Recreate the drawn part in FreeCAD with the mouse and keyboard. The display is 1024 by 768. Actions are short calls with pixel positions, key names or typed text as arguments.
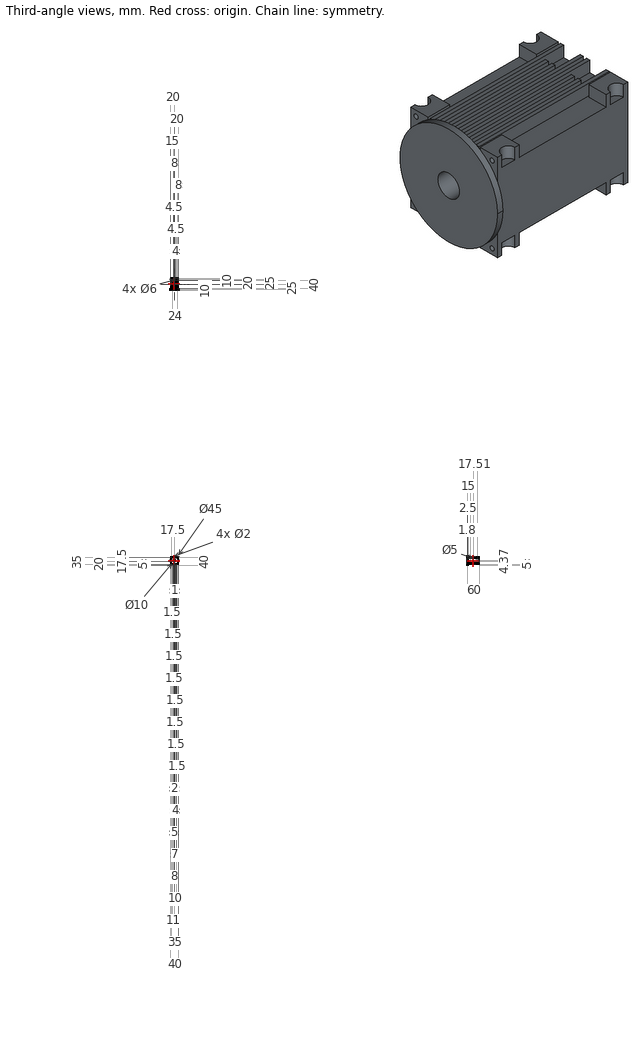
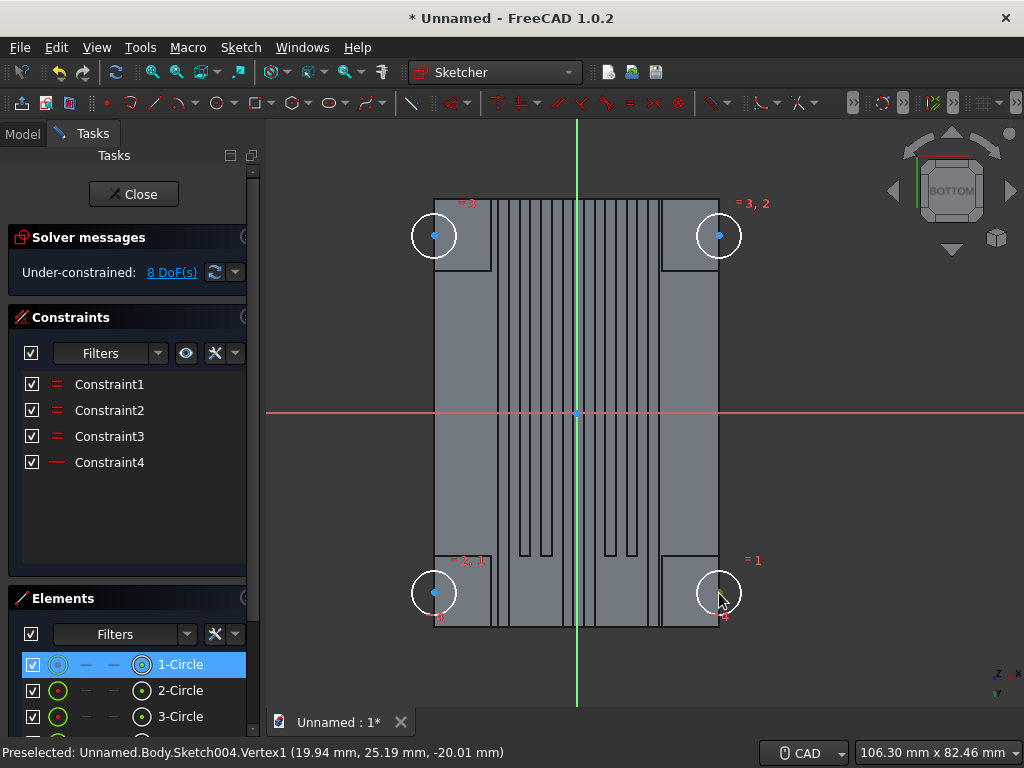
click(719, 236)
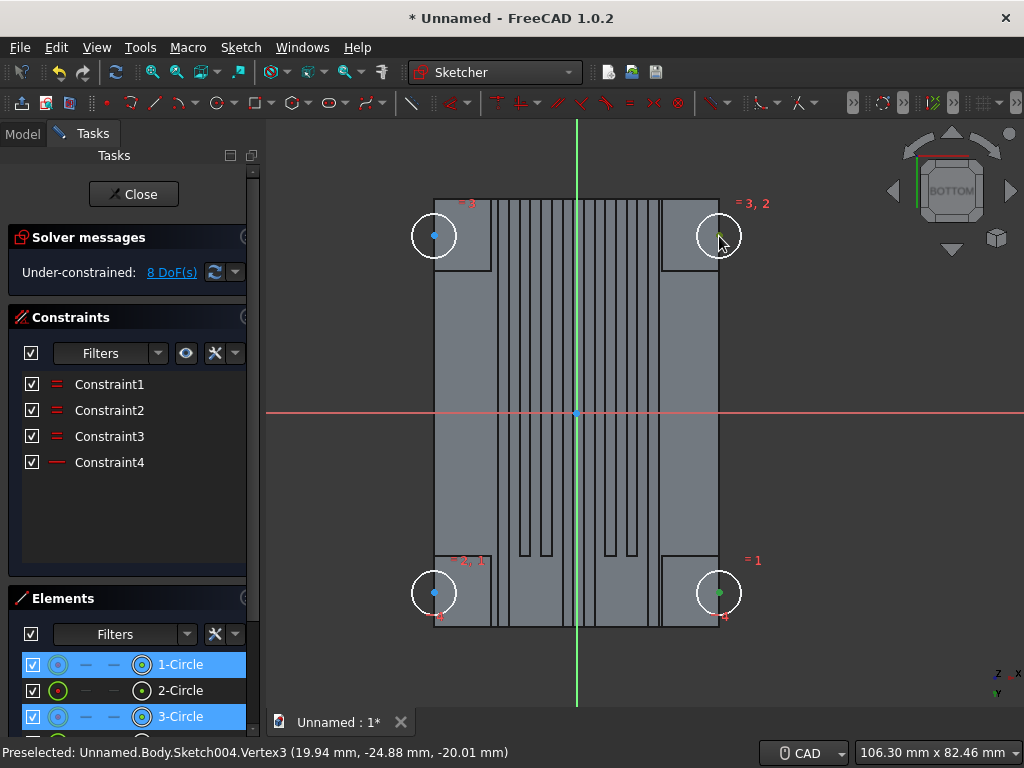
click(540, 104)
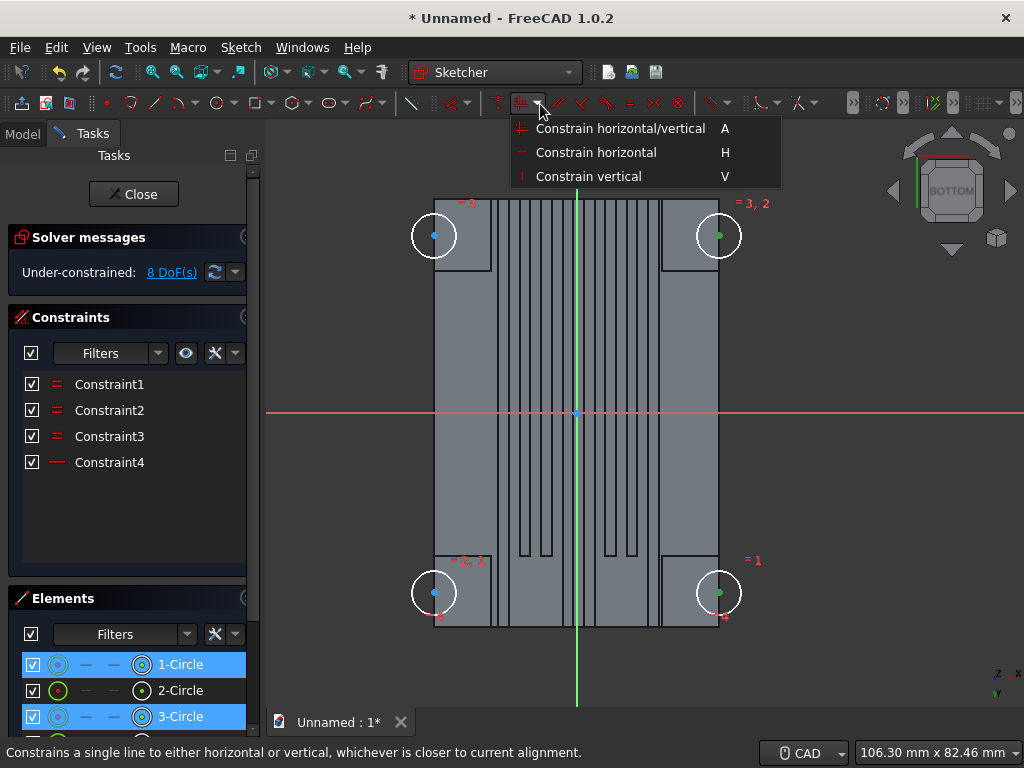
click(646, 176)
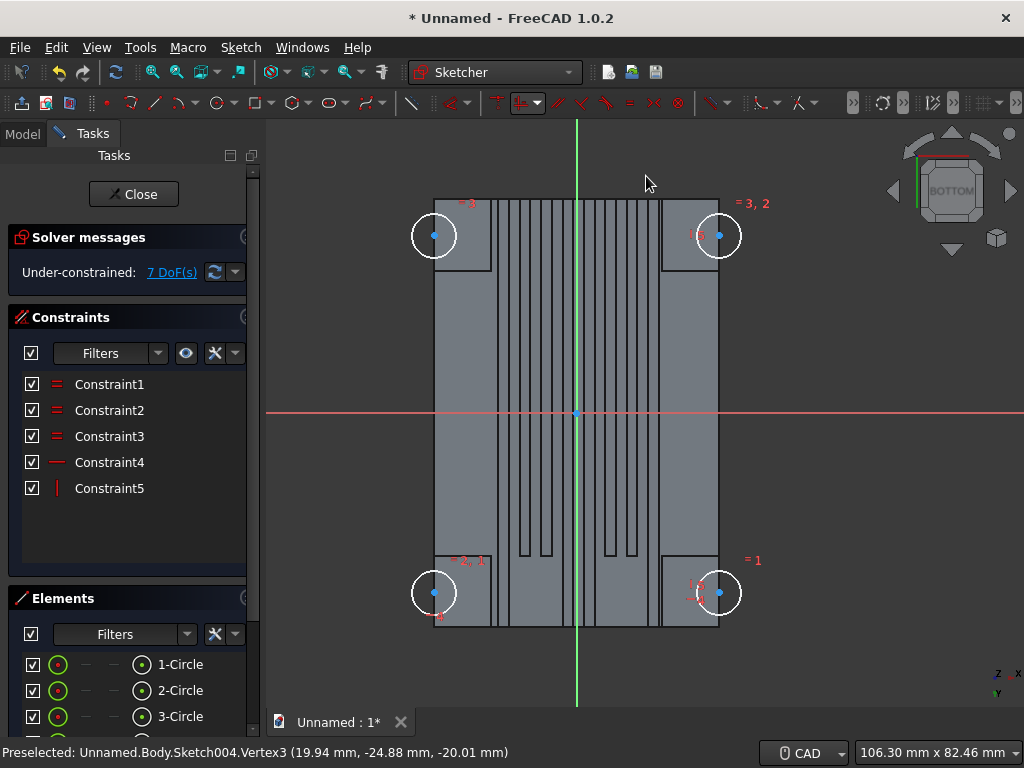
click(434, 593)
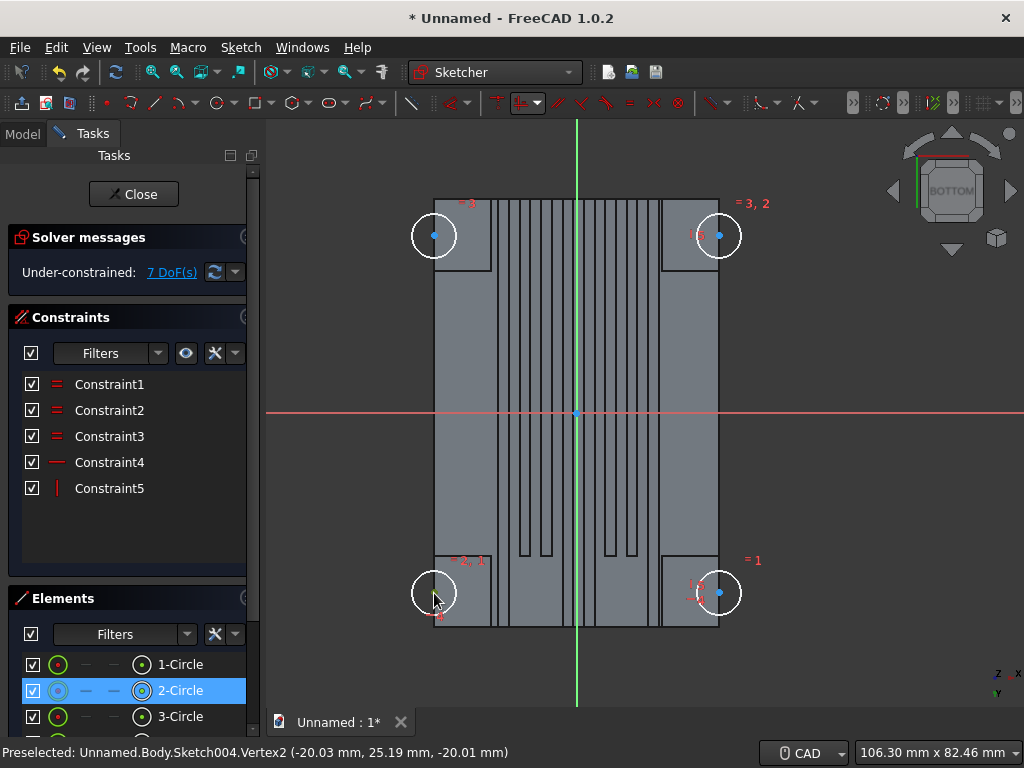
click(434, 236)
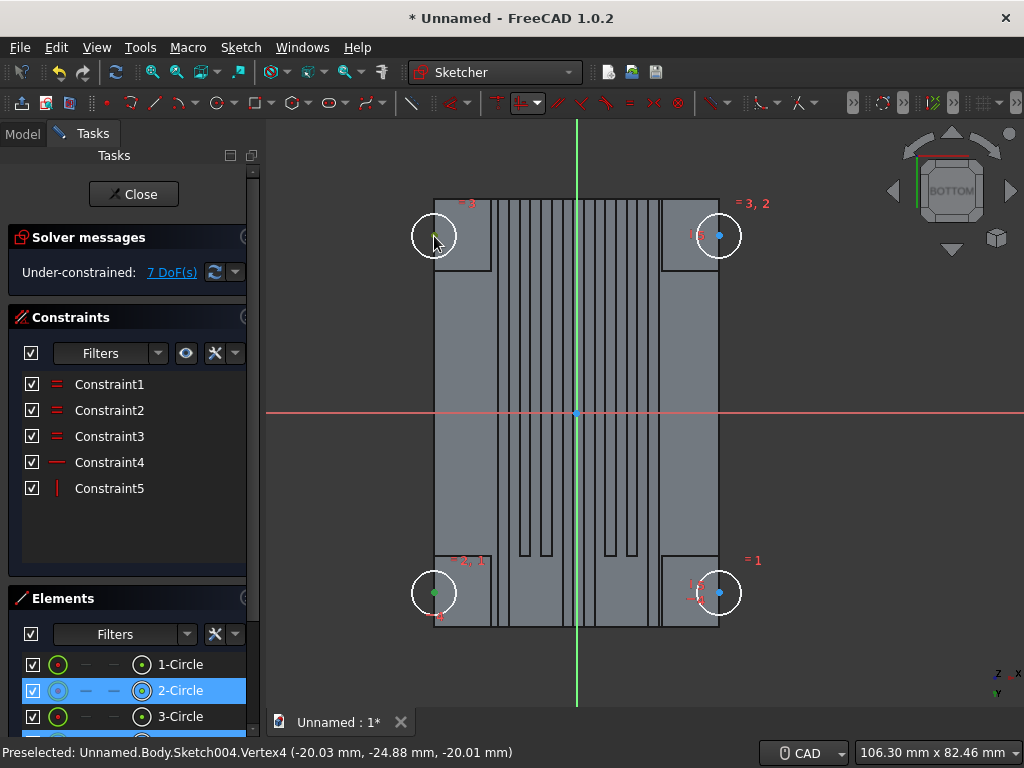
click(540, 104)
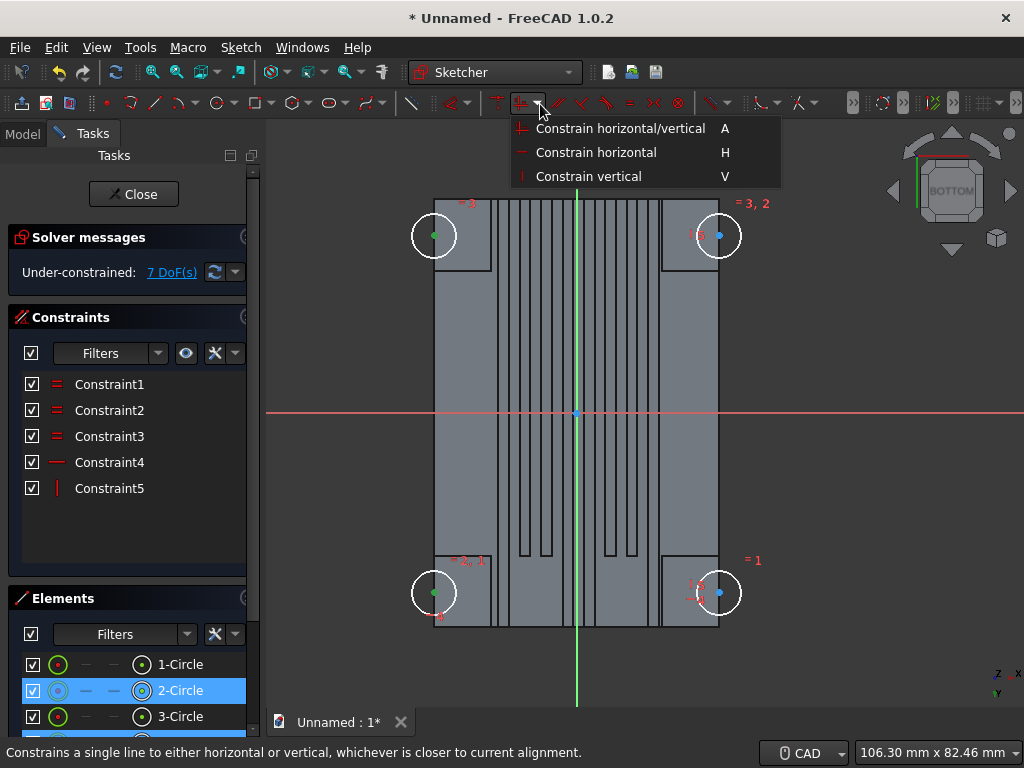
click(646, 176)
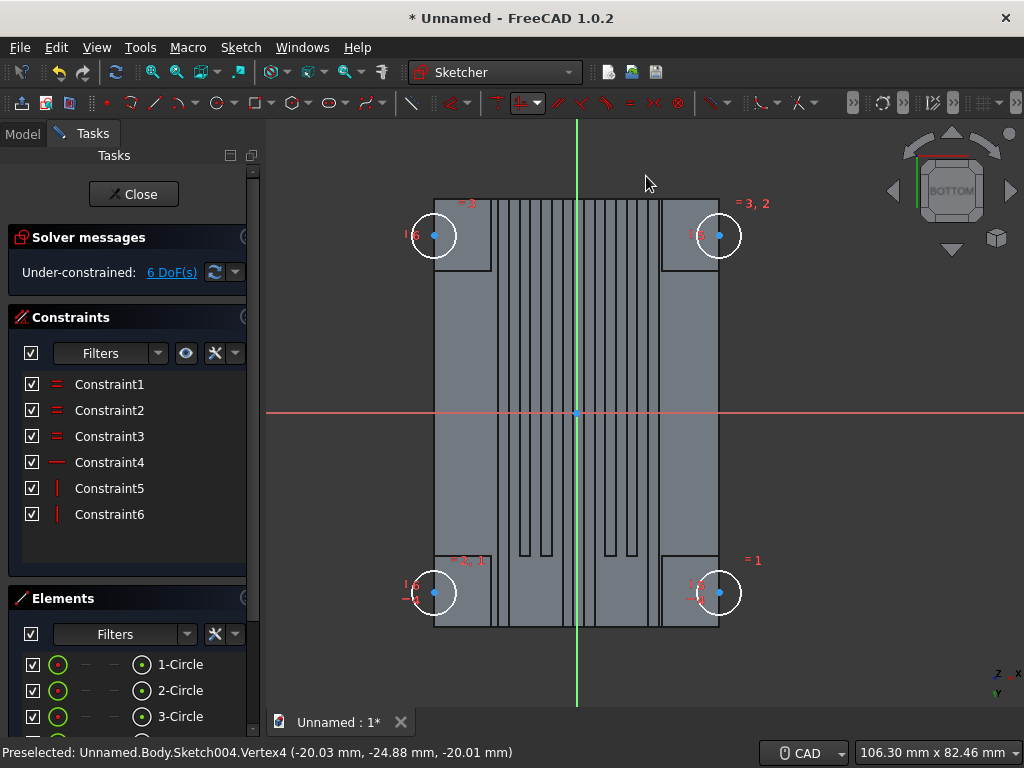
click(719, 236)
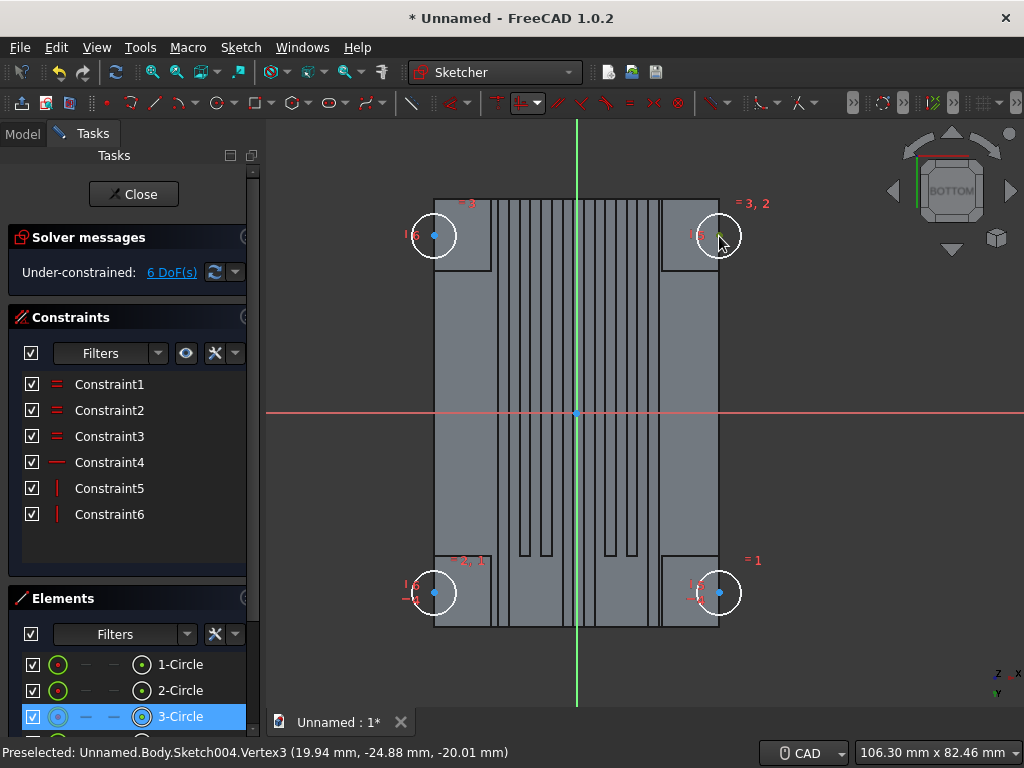
click(434, 236)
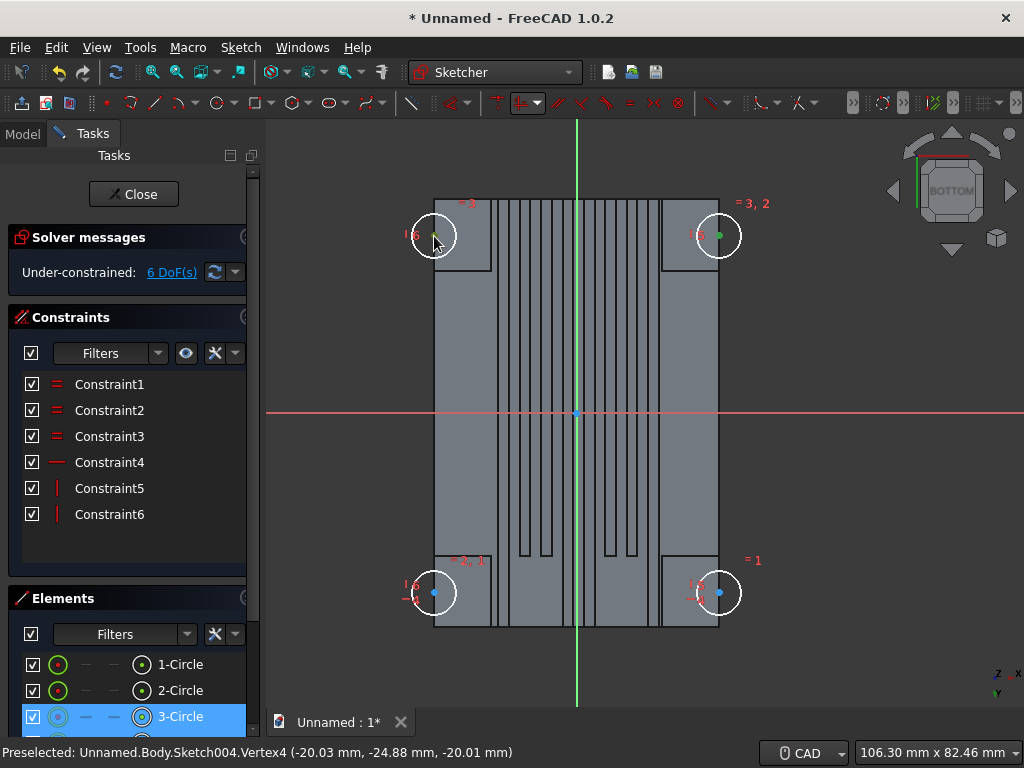
click(540, 104)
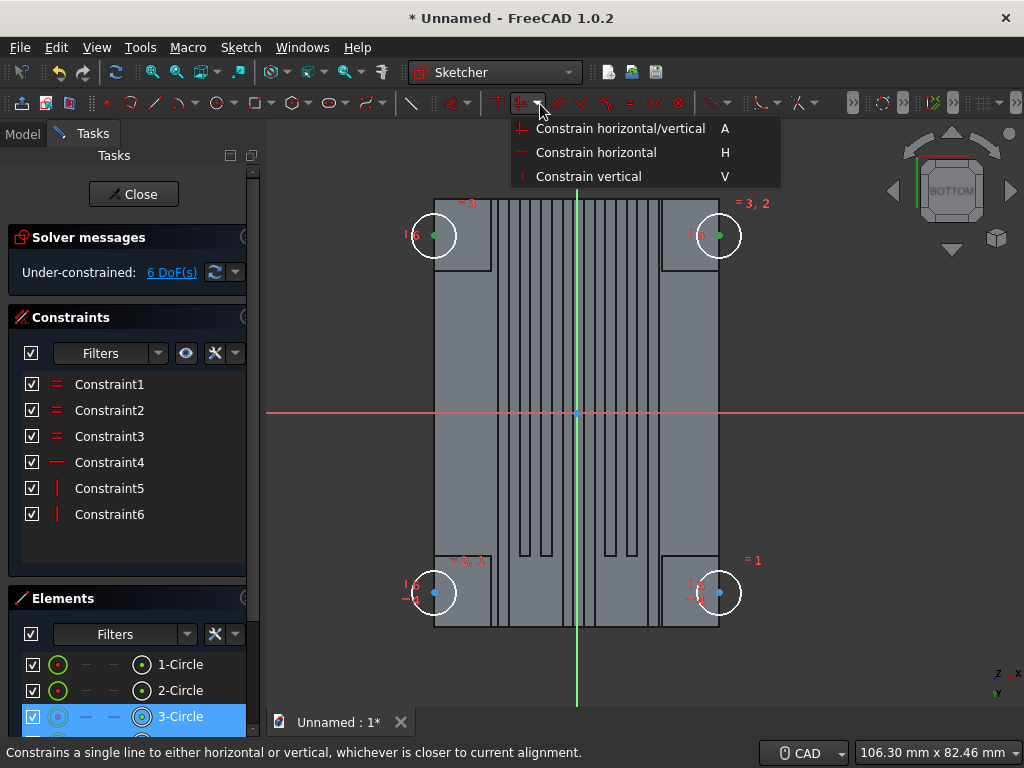
click(646, 152)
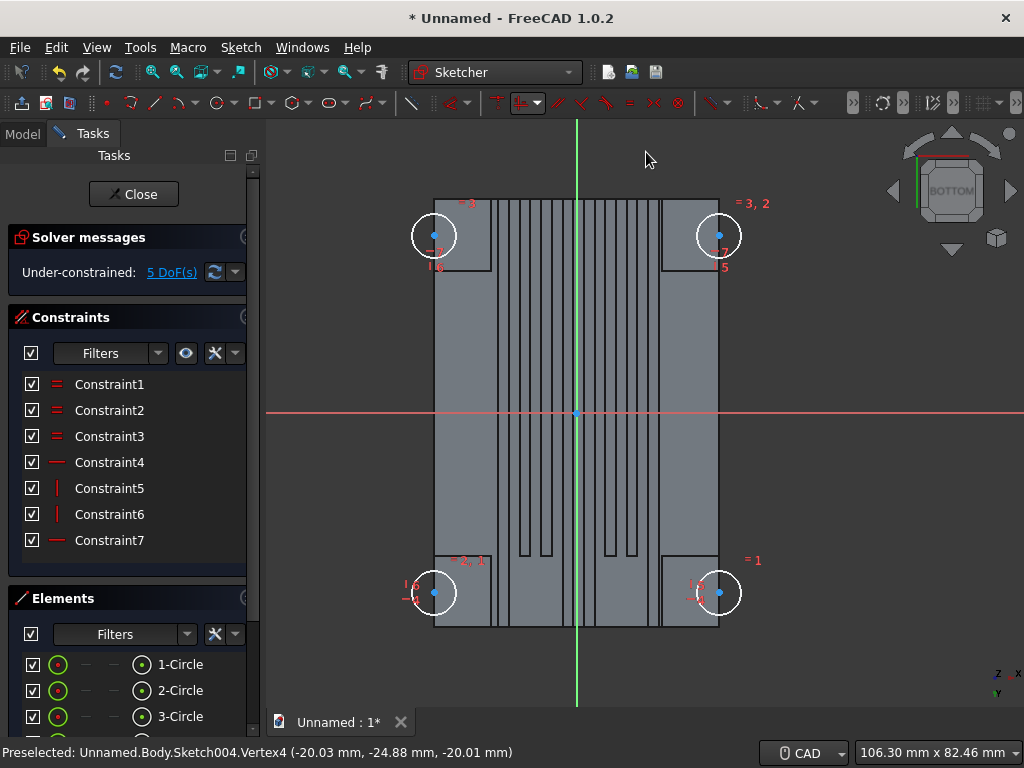
click(450, 104)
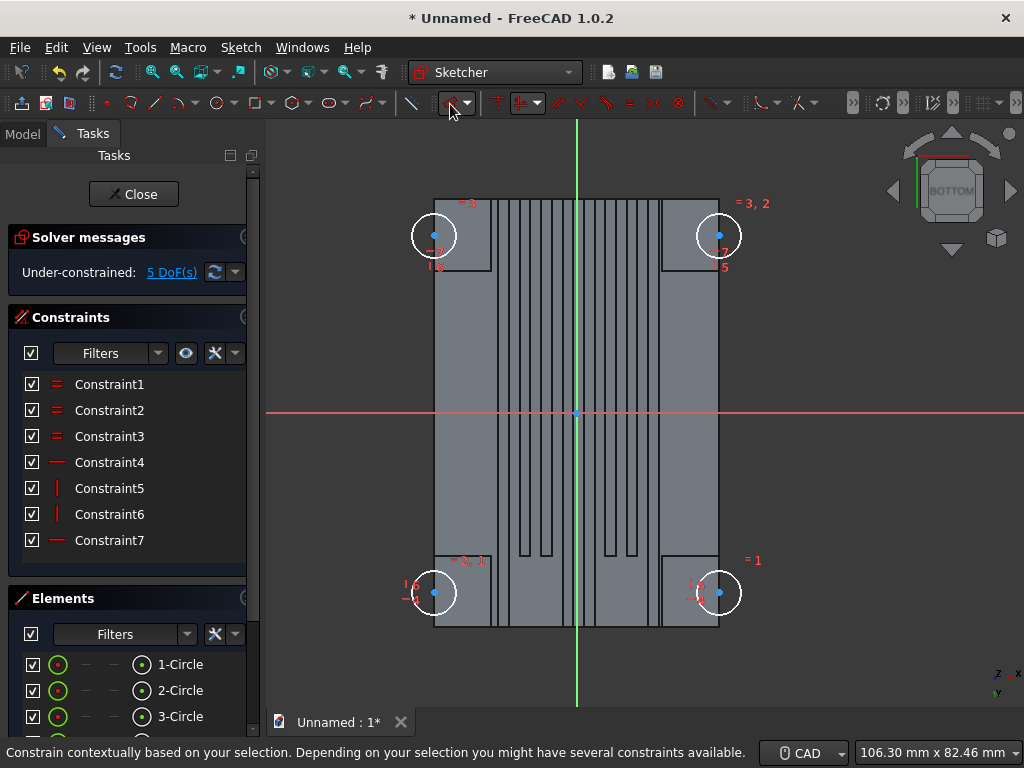
click(734, 577)
click(756, 554)